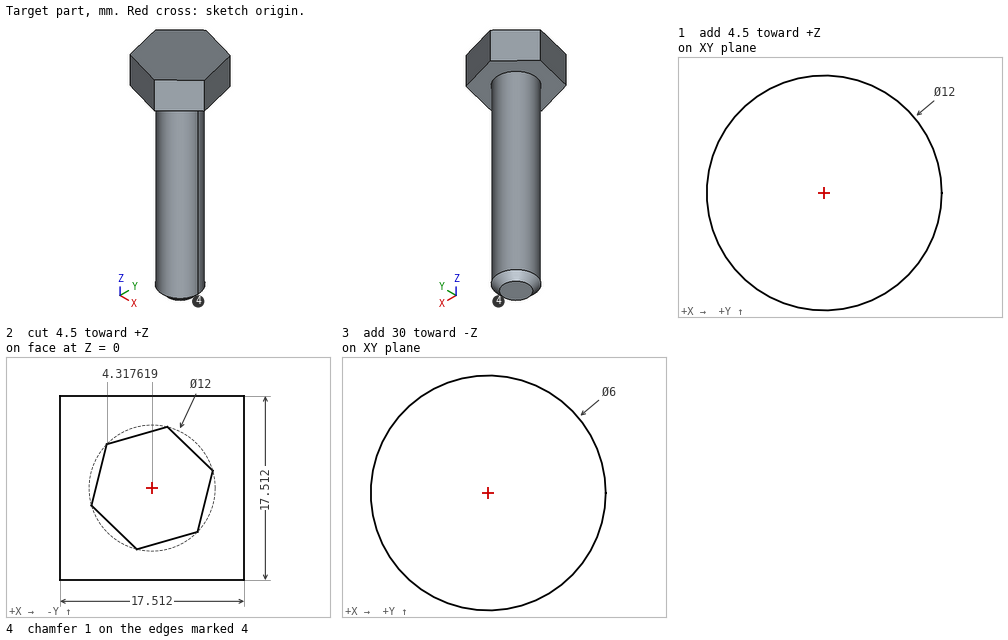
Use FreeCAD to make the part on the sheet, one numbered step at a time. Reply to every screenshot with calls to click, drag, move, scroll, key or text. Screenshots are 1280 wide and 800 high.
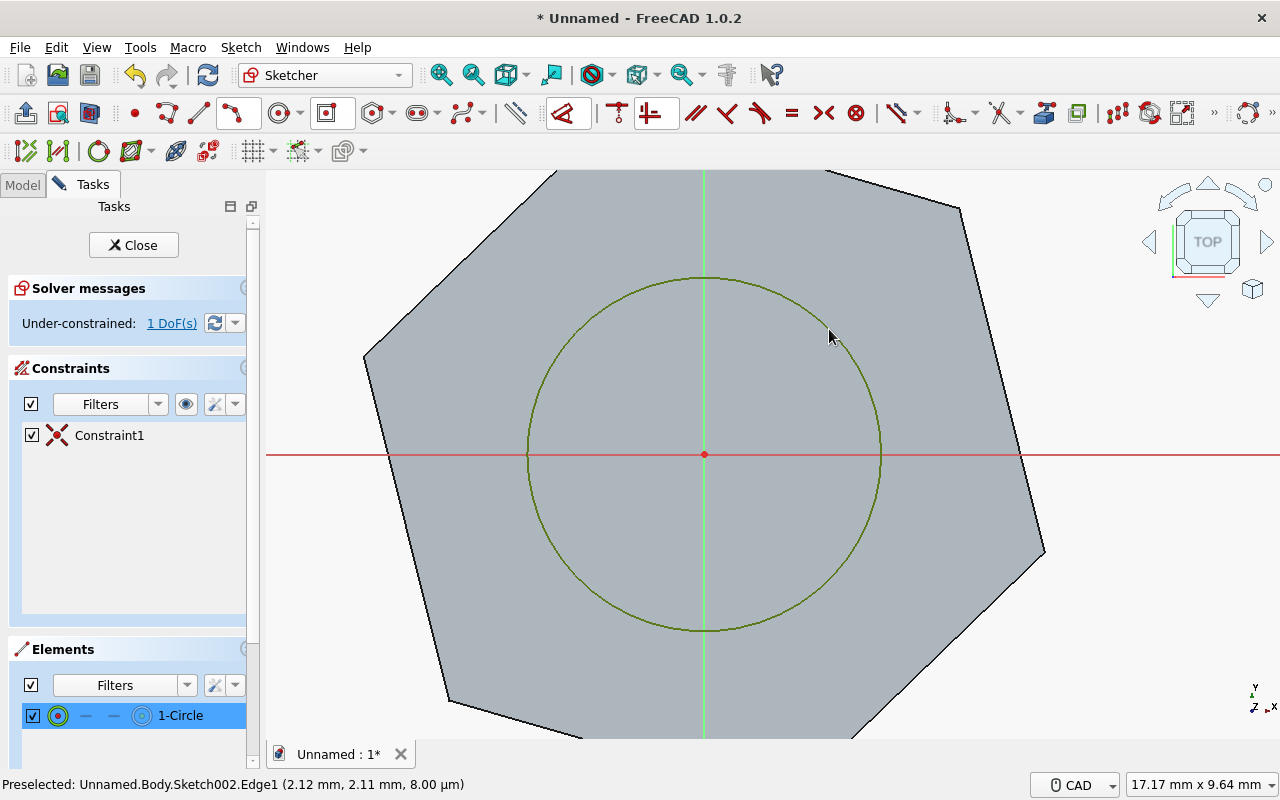
key(k)
key(o)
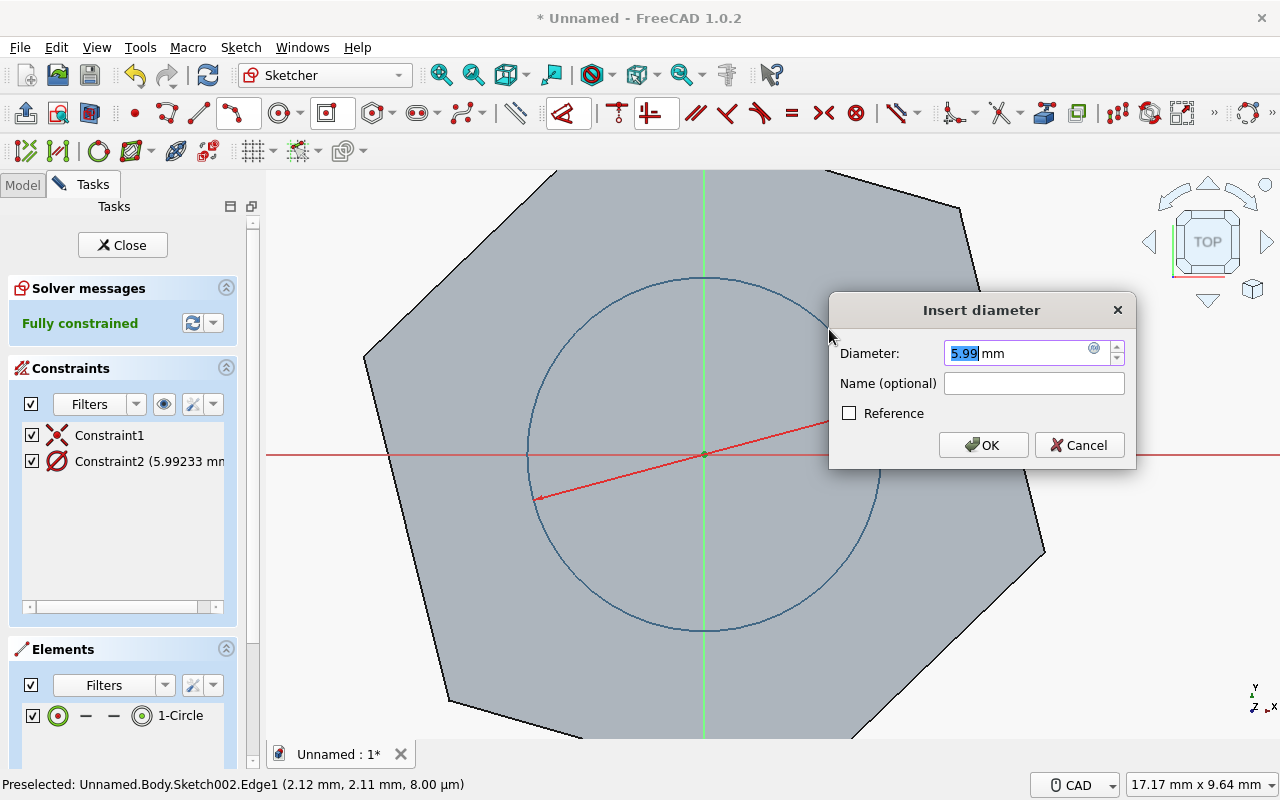
text(6)
key(Return)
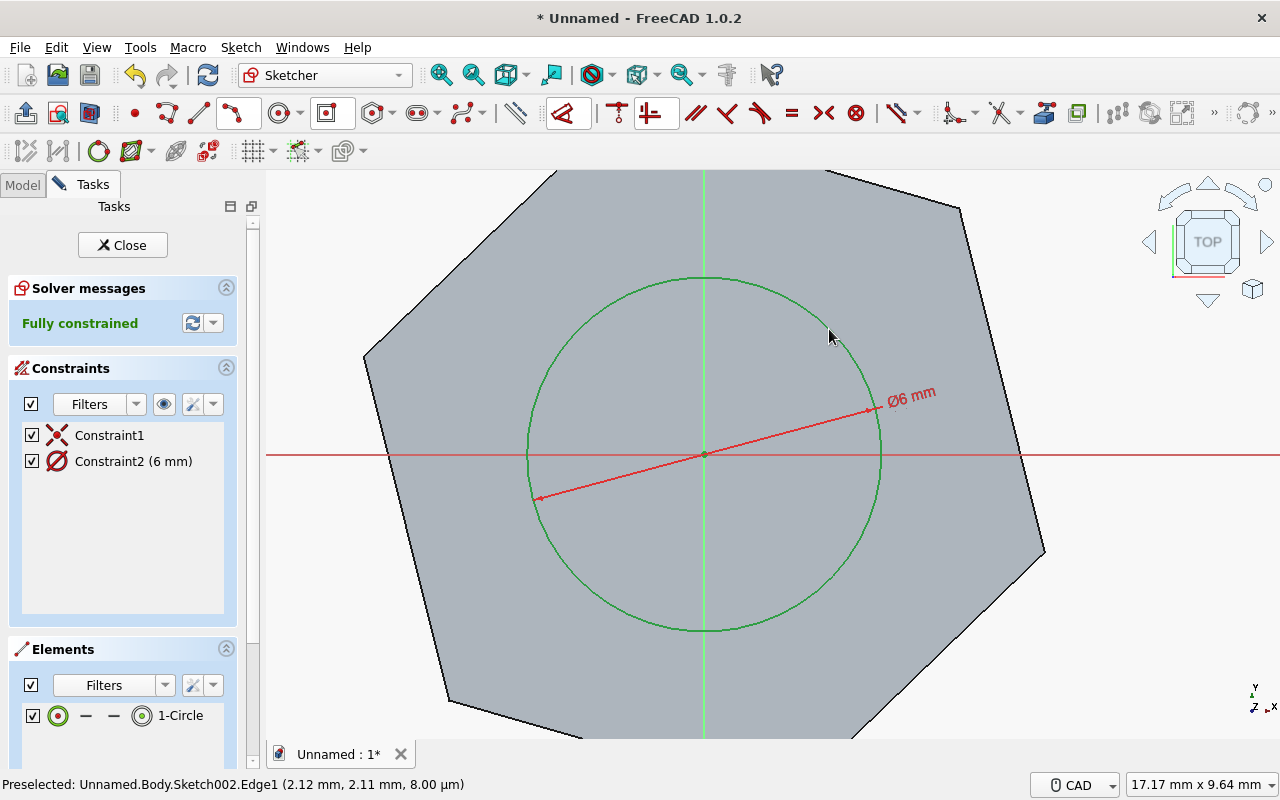
click(123, 245)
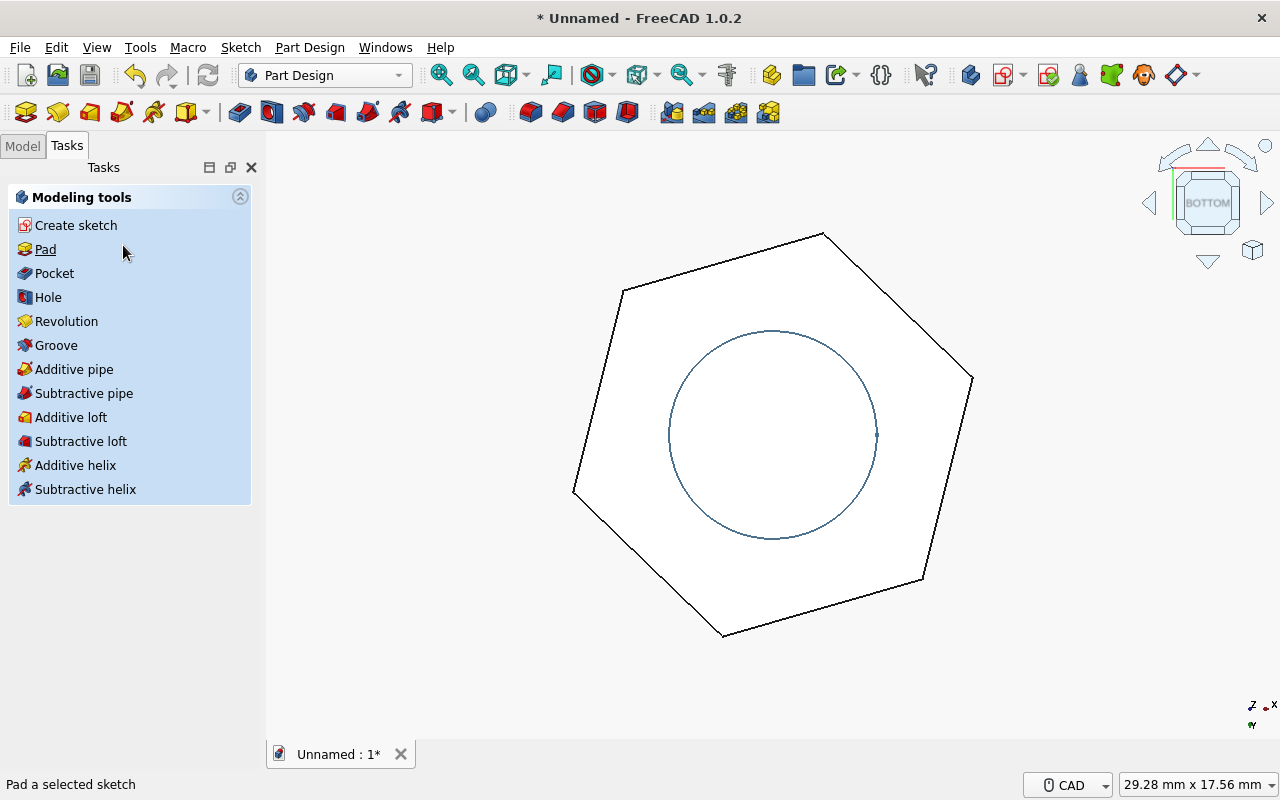
click(26, 112)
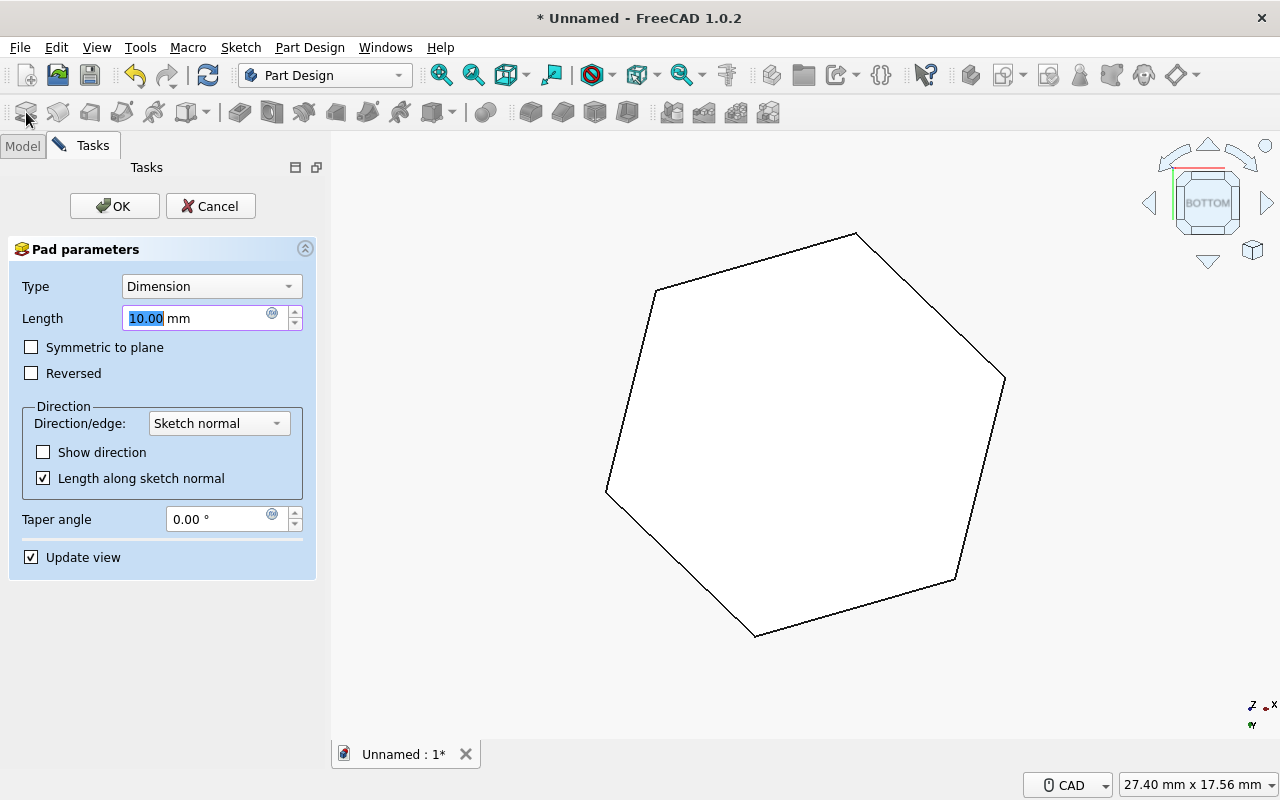
text(30)
key(Tab)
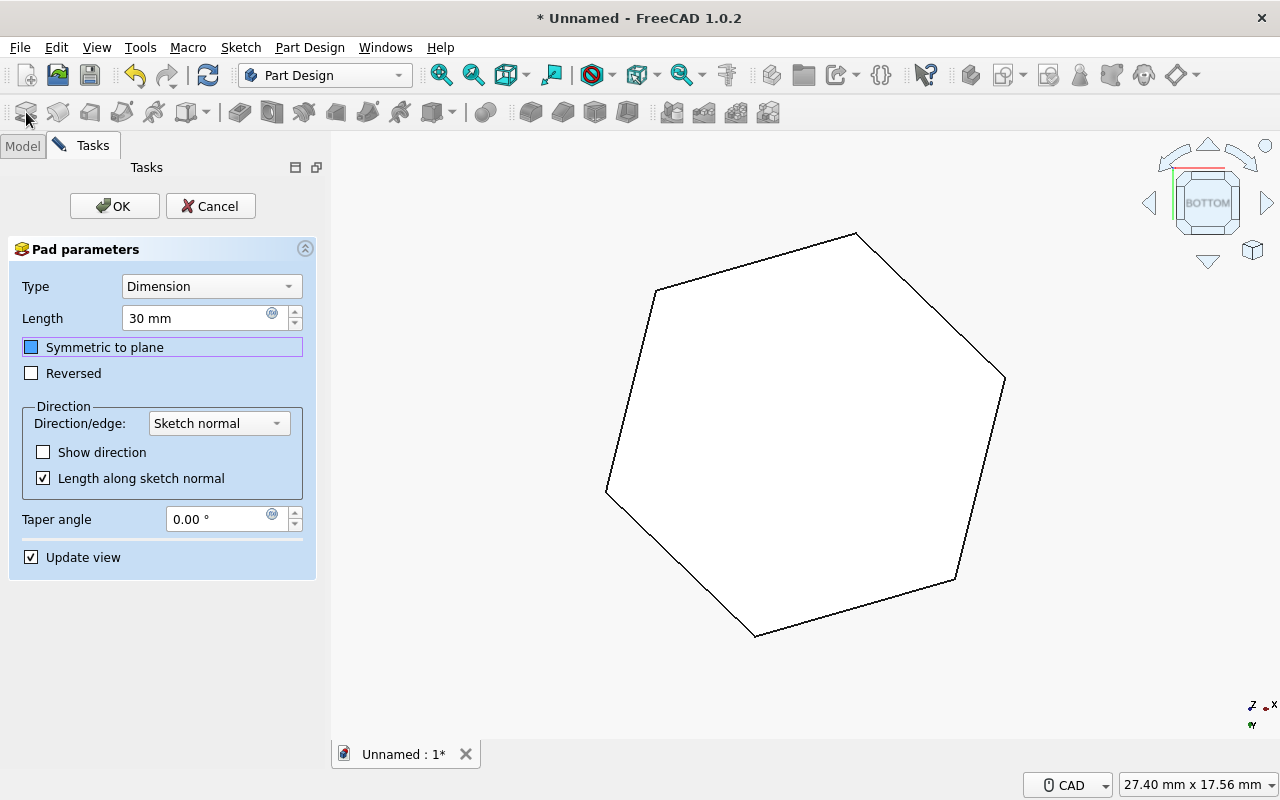
click(30, 373)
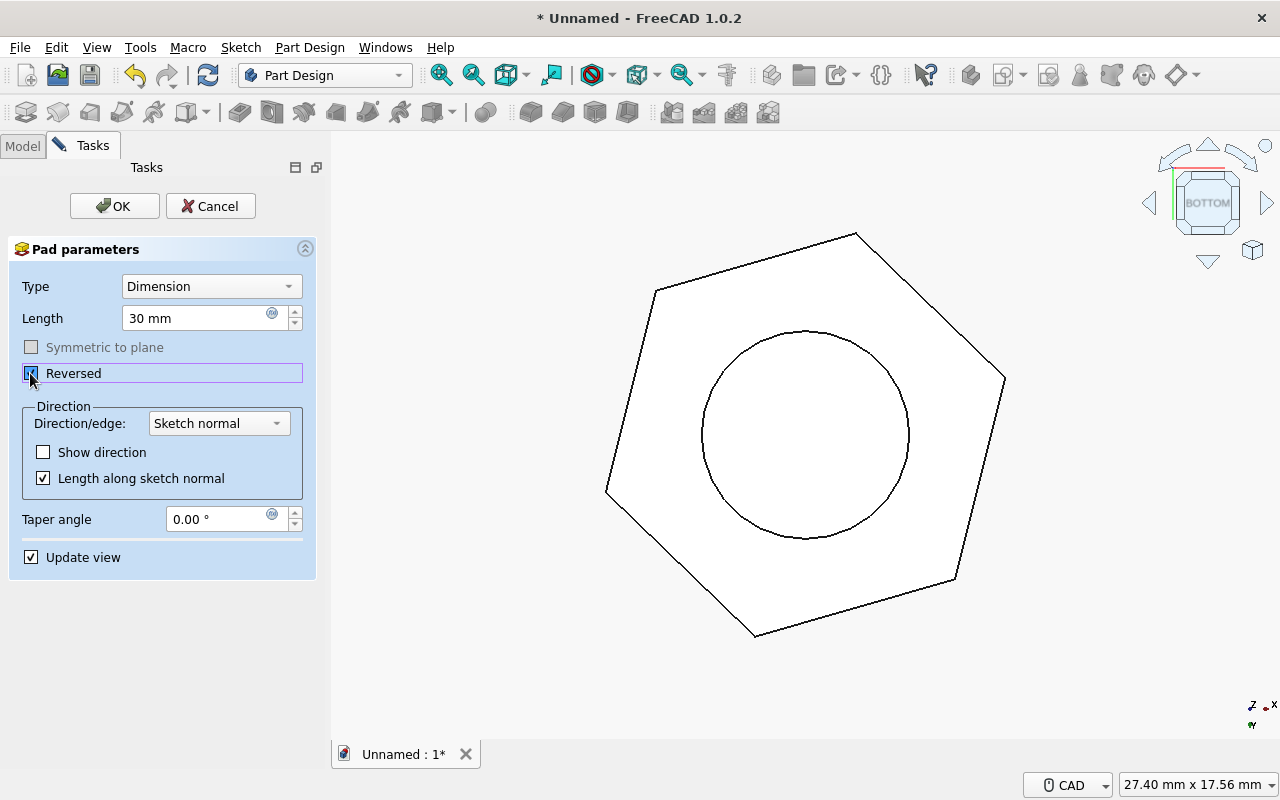
click(115, 206)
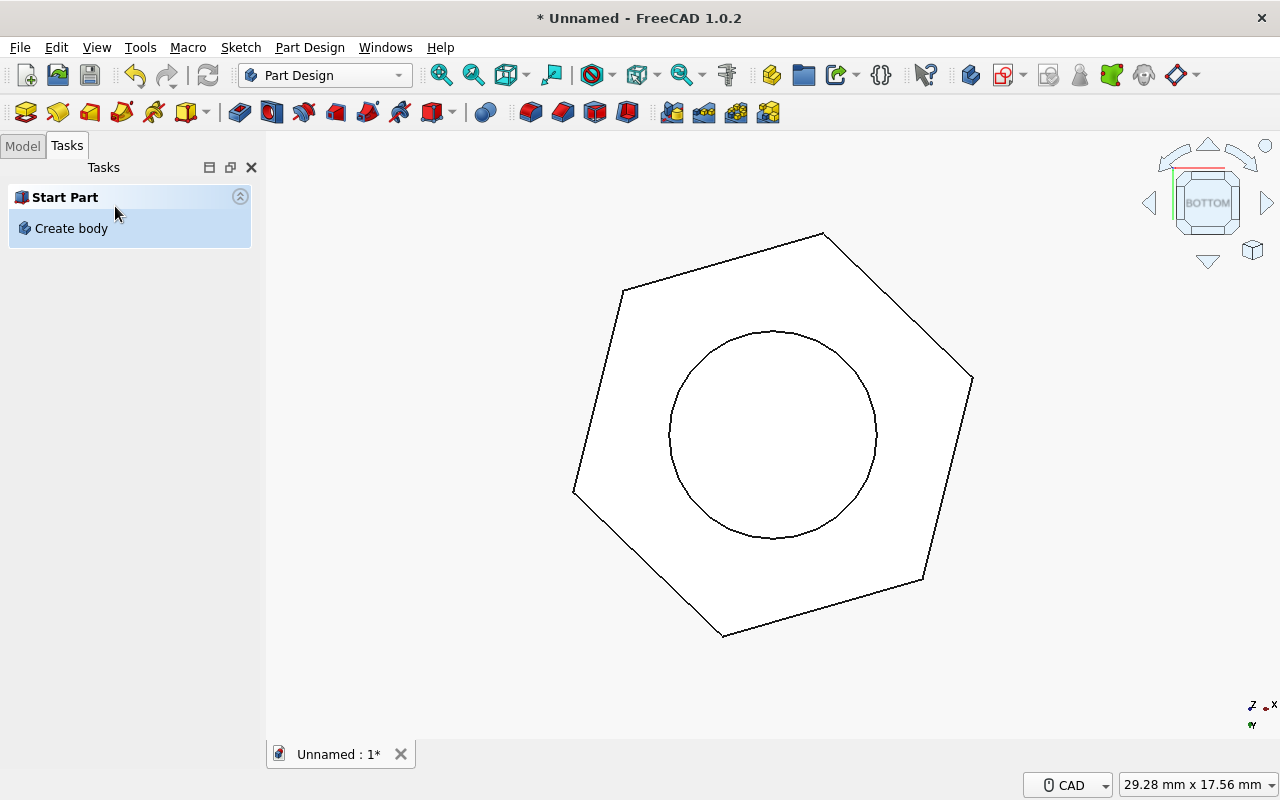
click(669, 434)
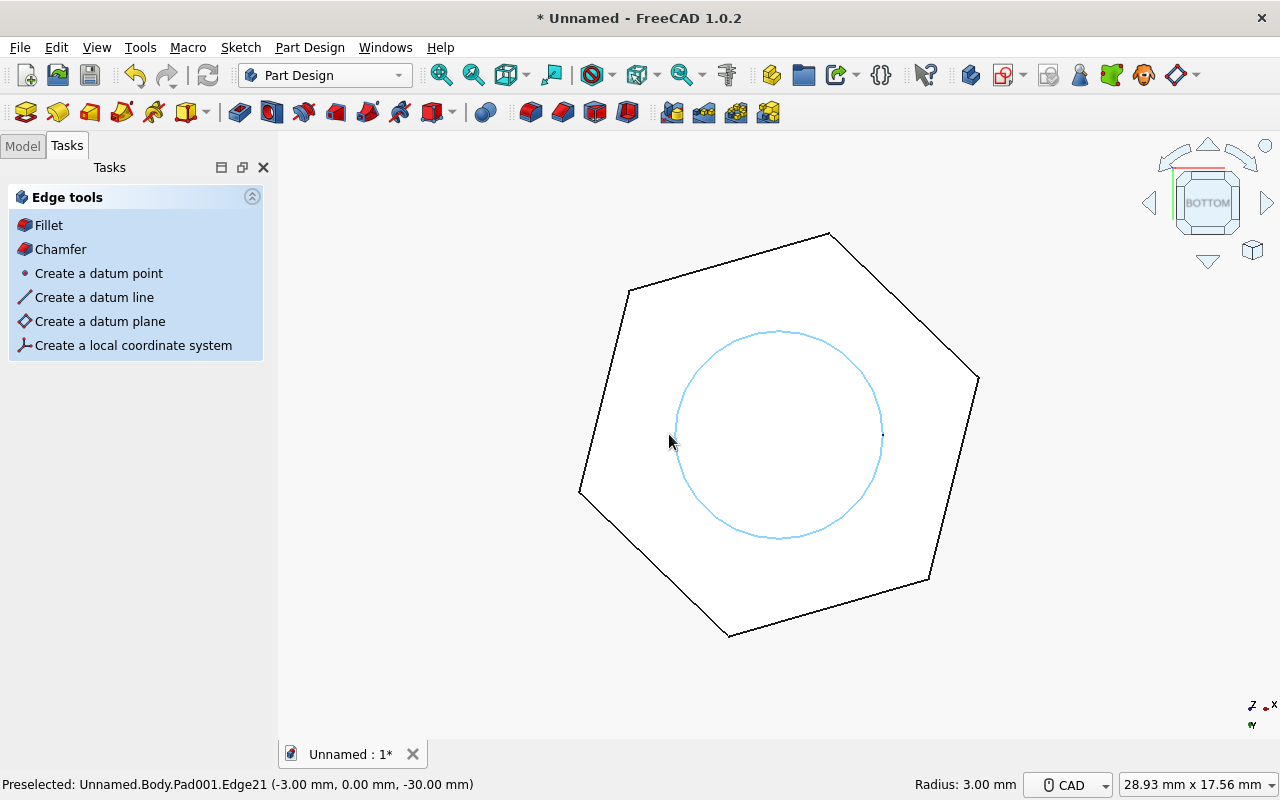
click(564, 112)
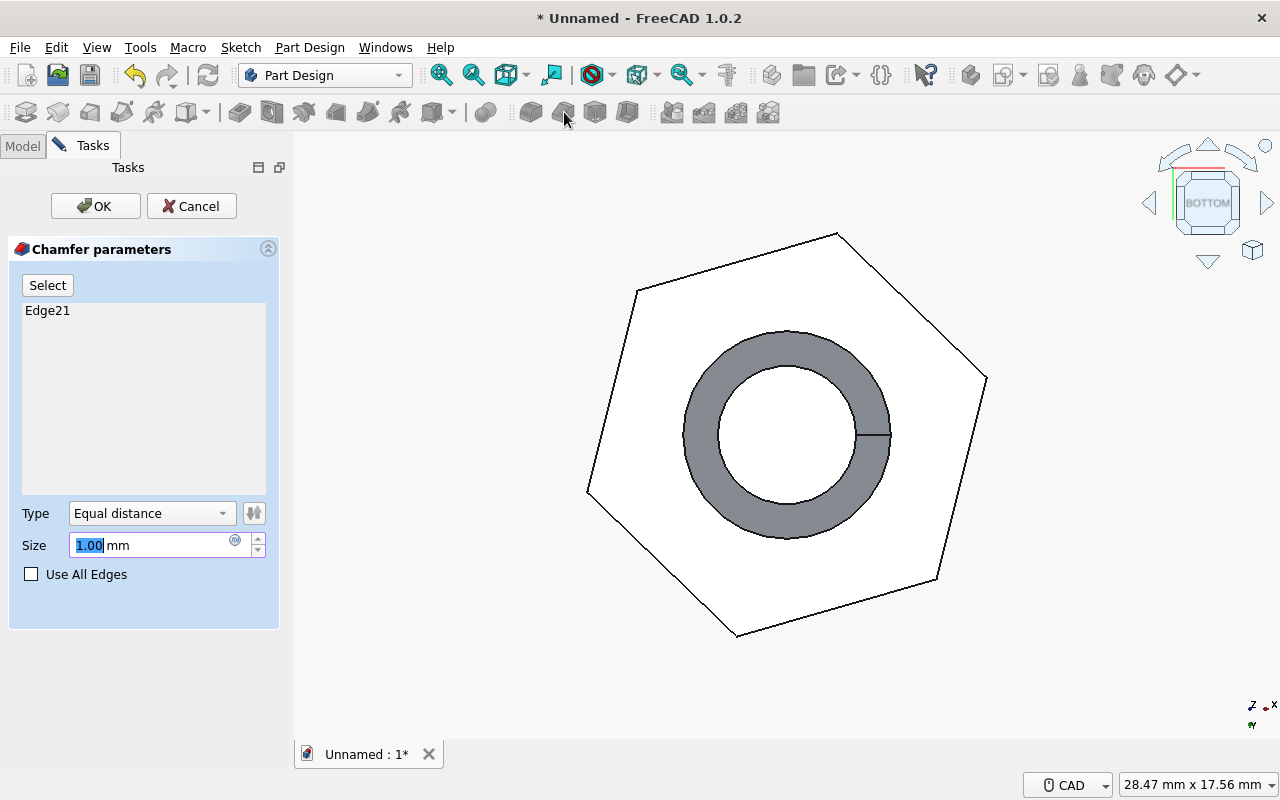
text(1)
key(Tab)